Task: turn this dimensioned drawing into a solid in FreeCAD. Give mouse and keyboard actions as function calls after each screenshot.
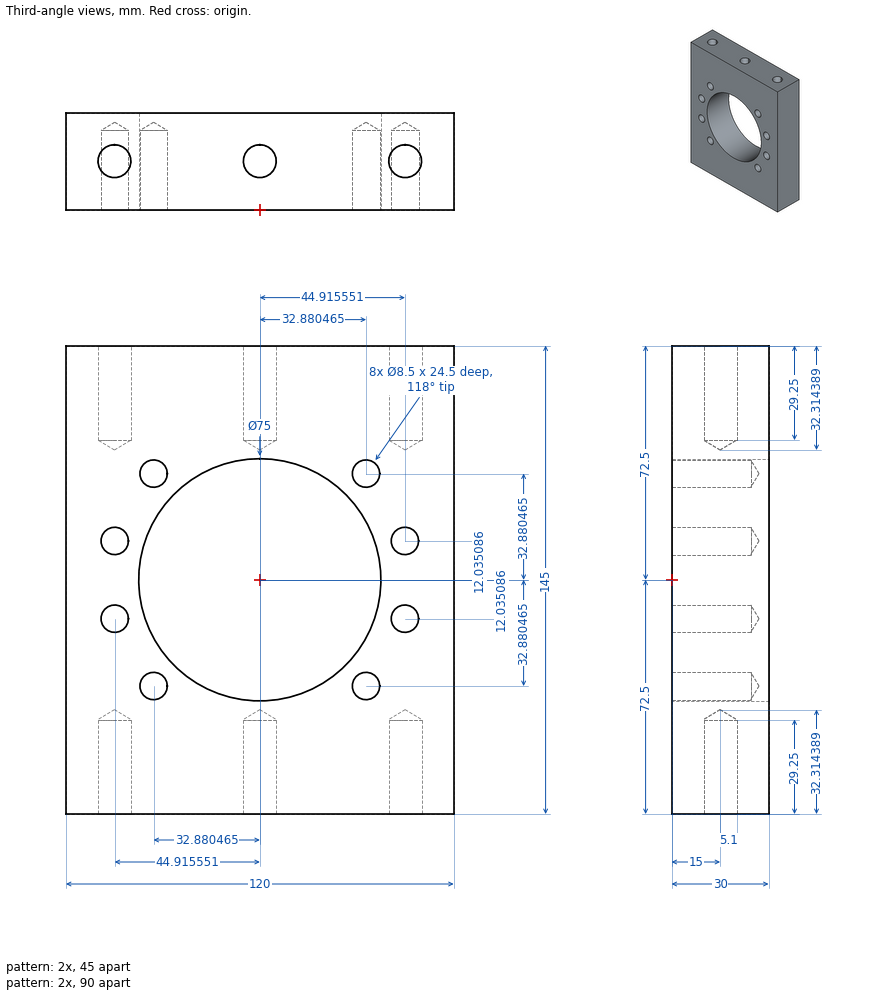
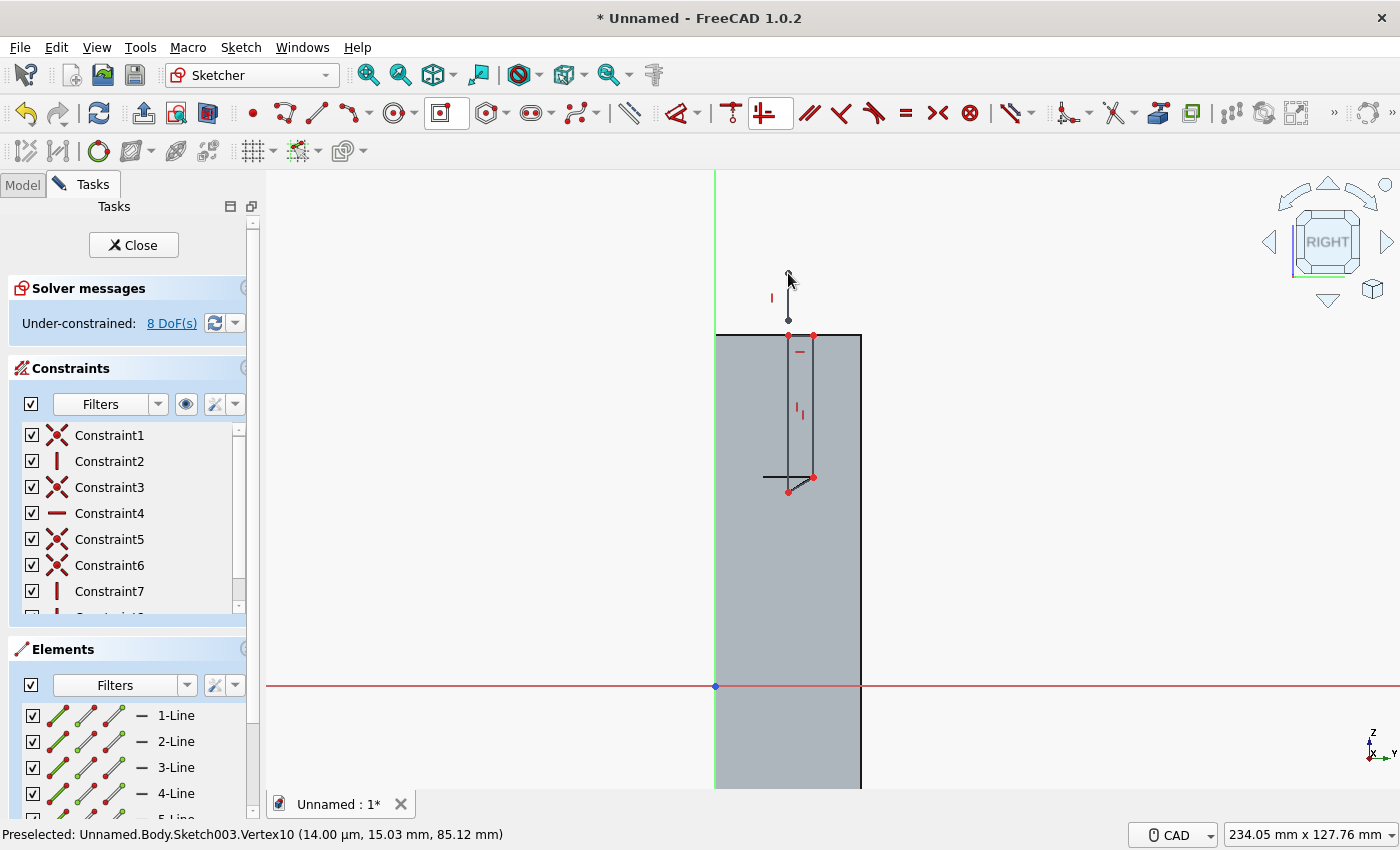
click(788, 307)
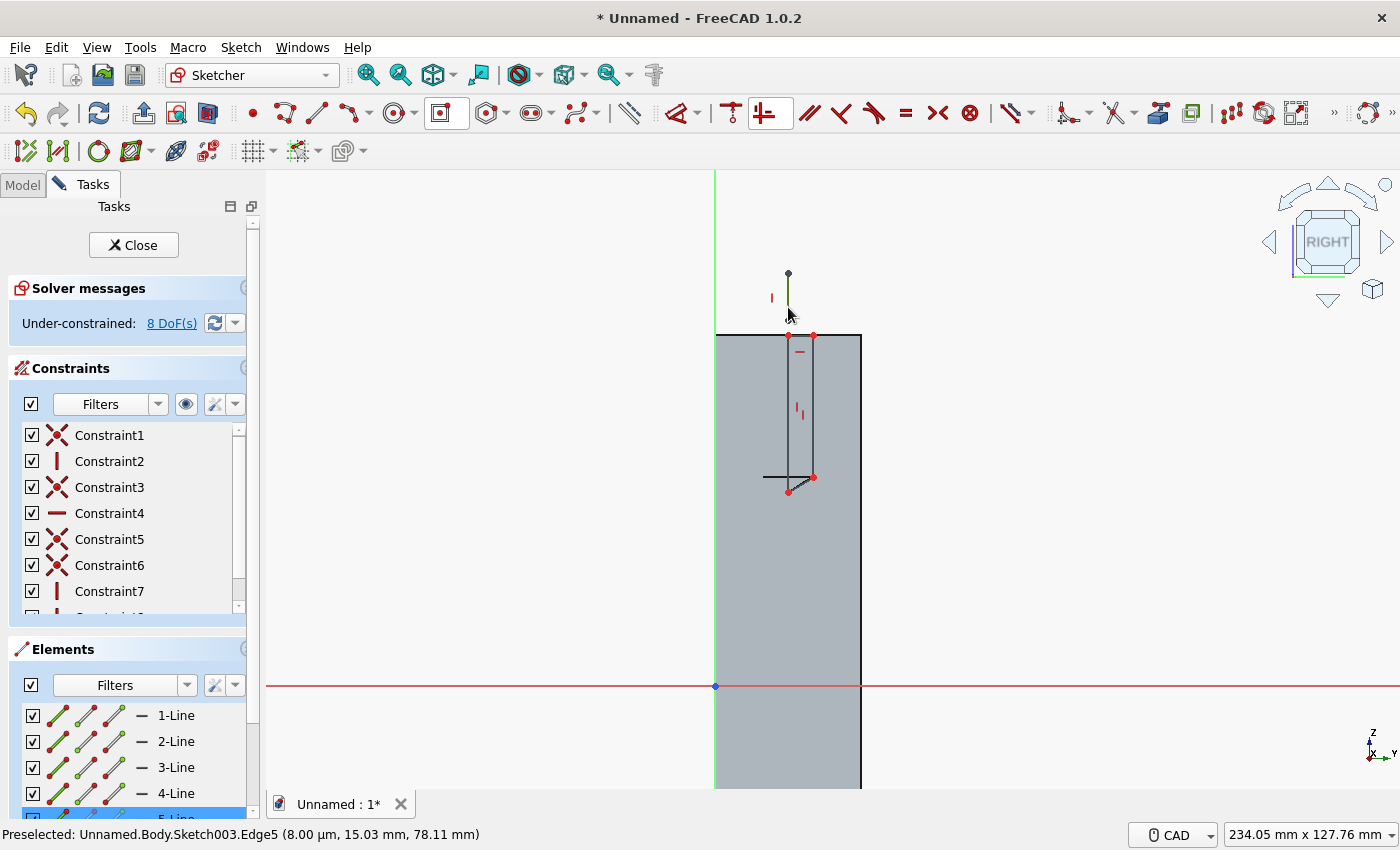
click(630, 114)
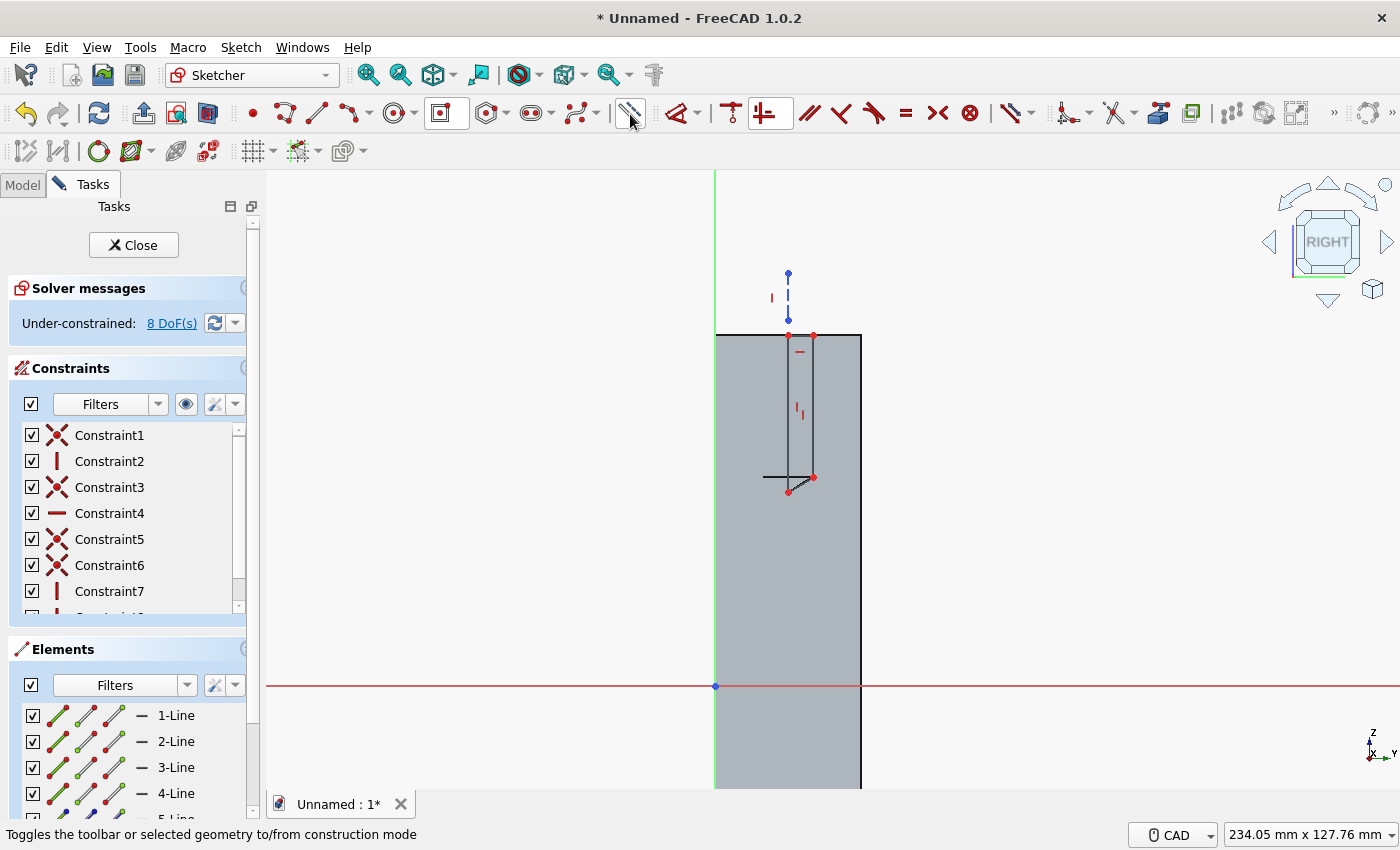
click(676, 114)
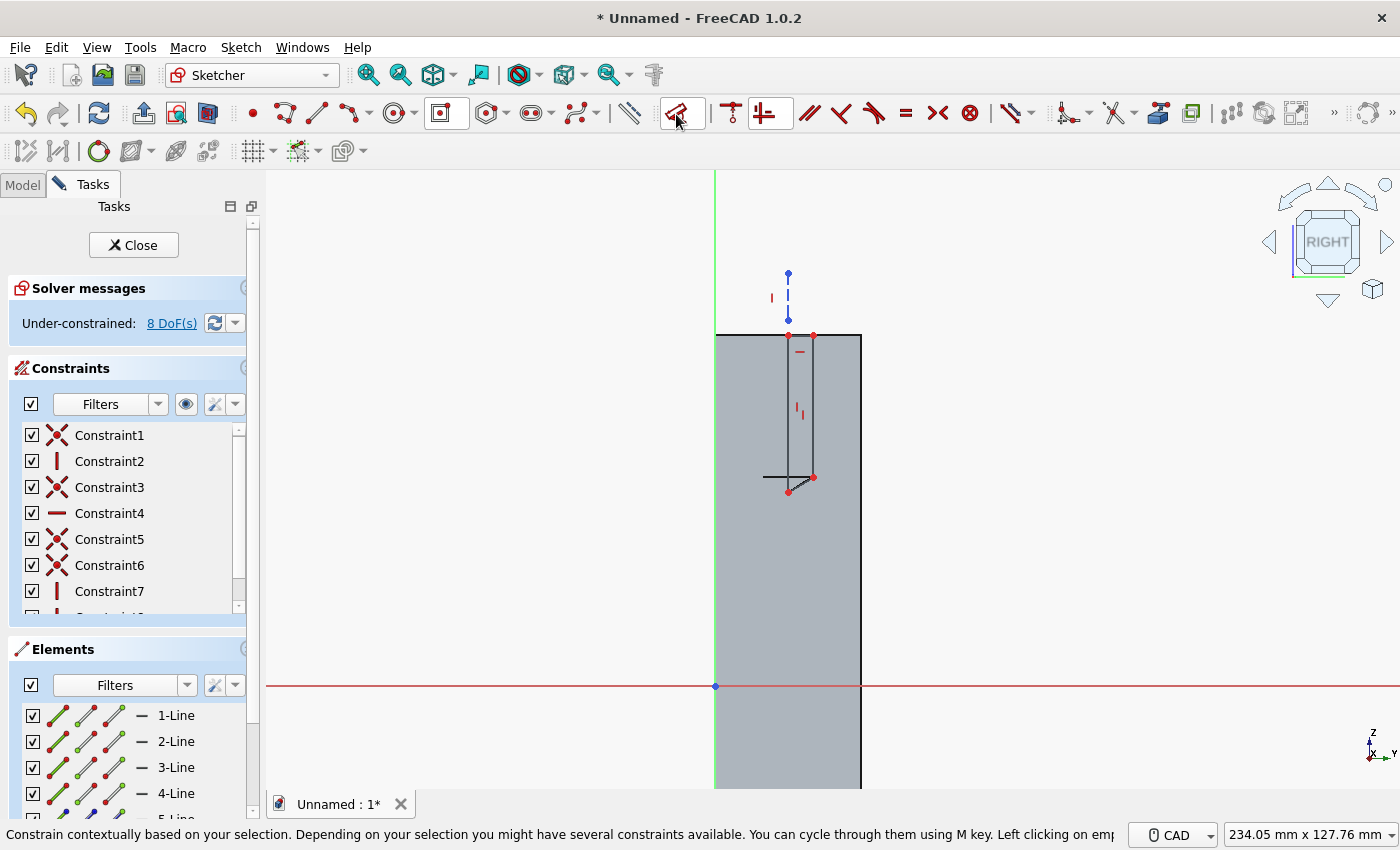
scroll(803, 336, up, 3)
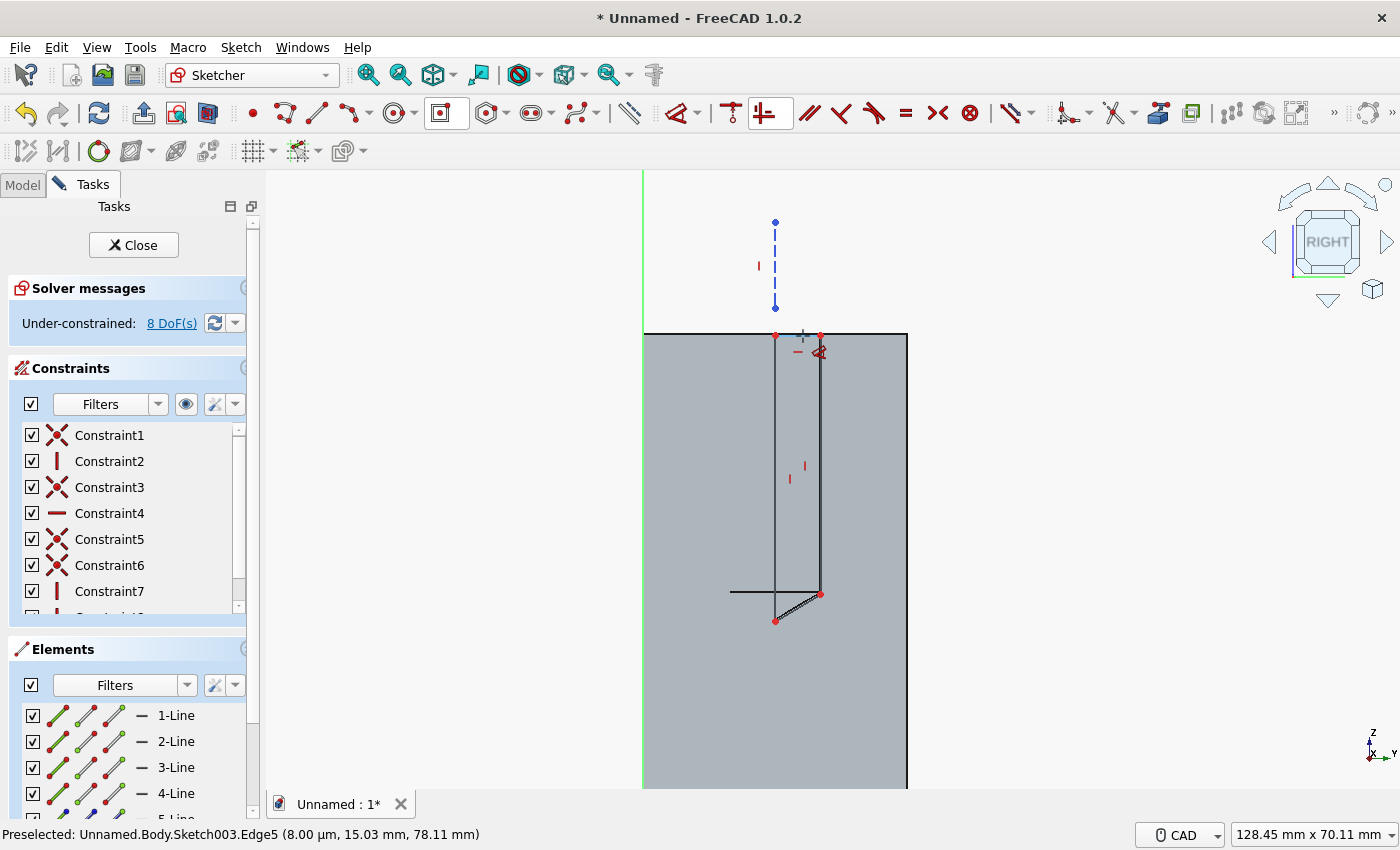
click(803, 336)
click(798, 302)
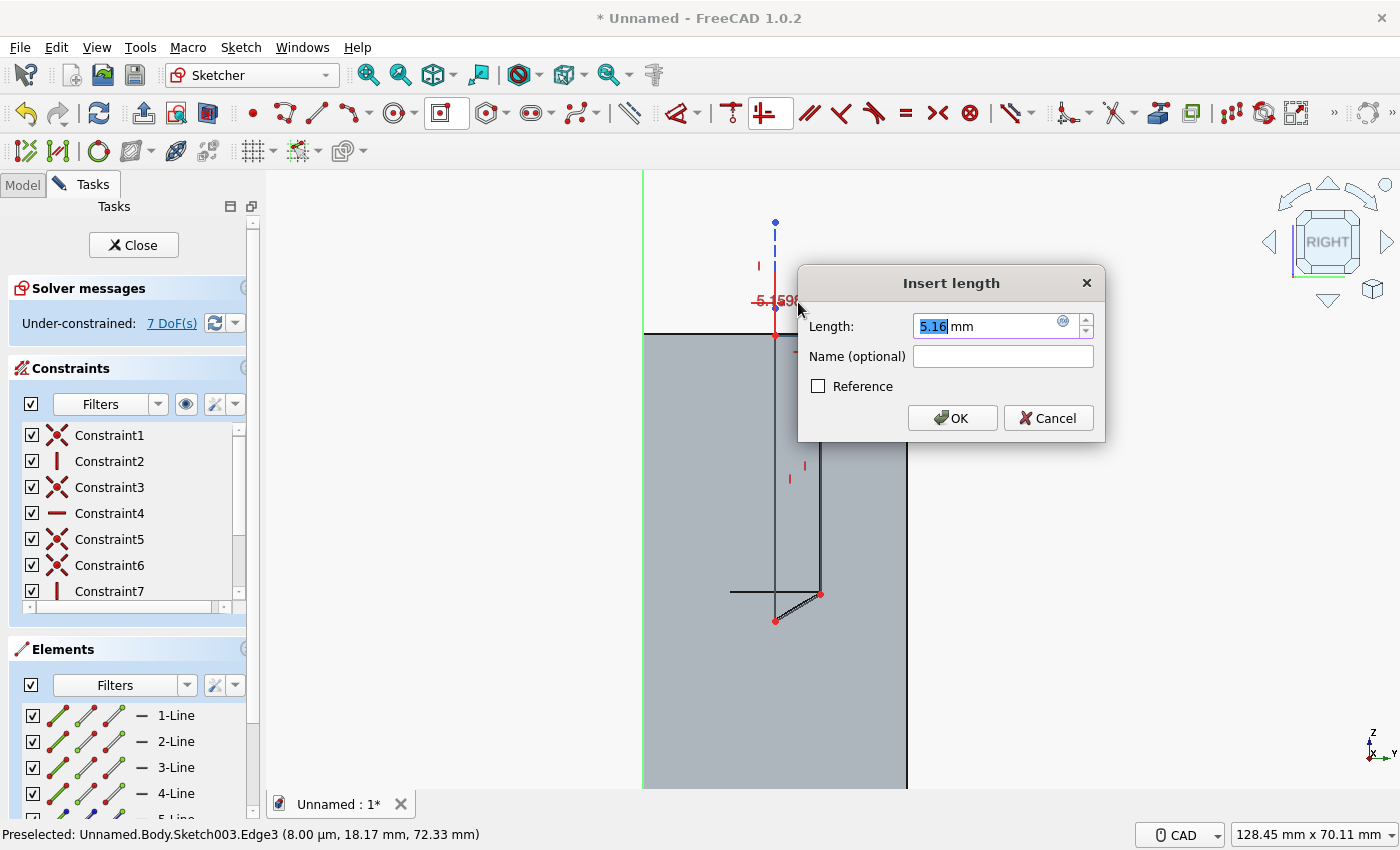
text(5.1)
key(Return)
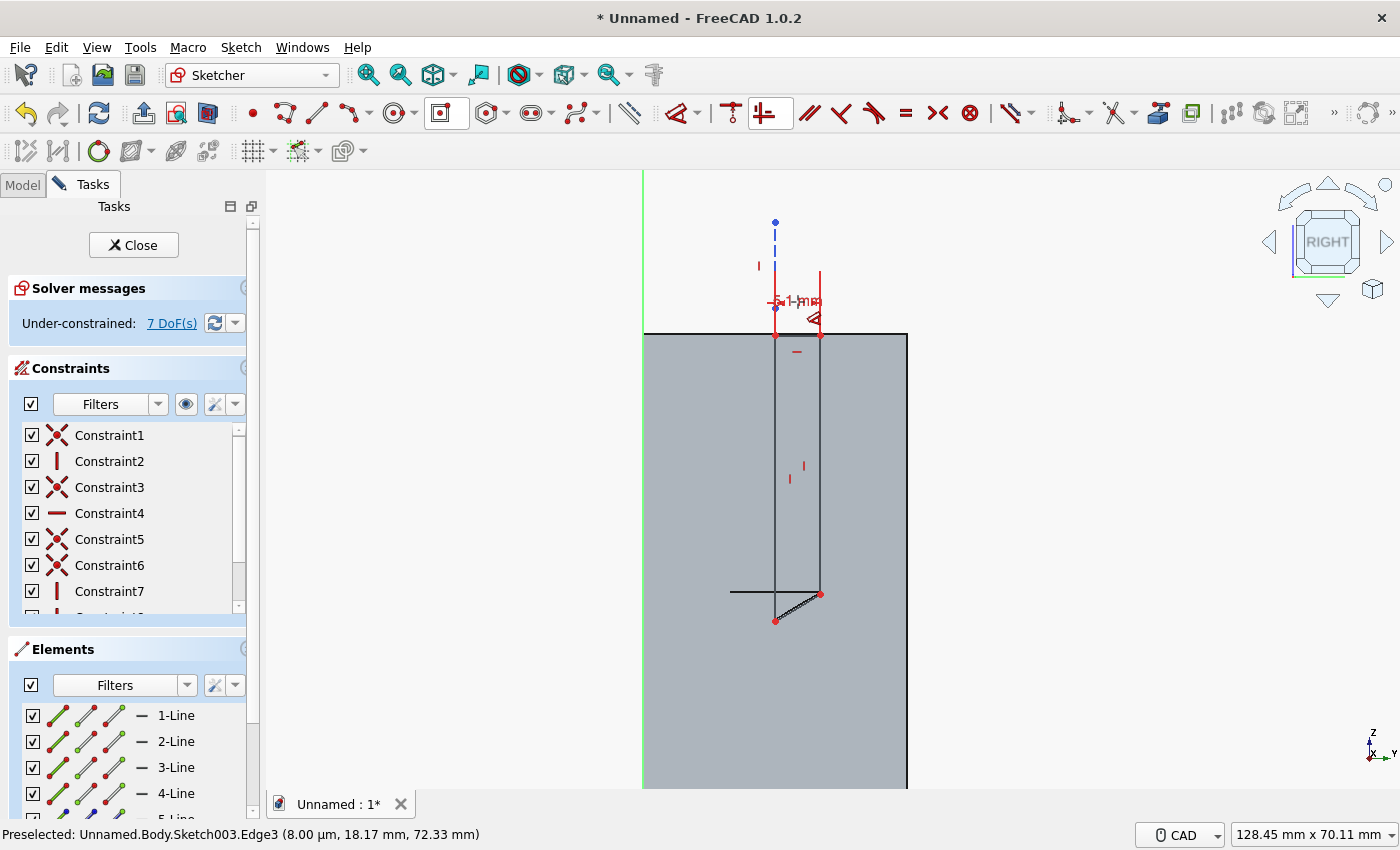
click(775, 622)
click(709, 588)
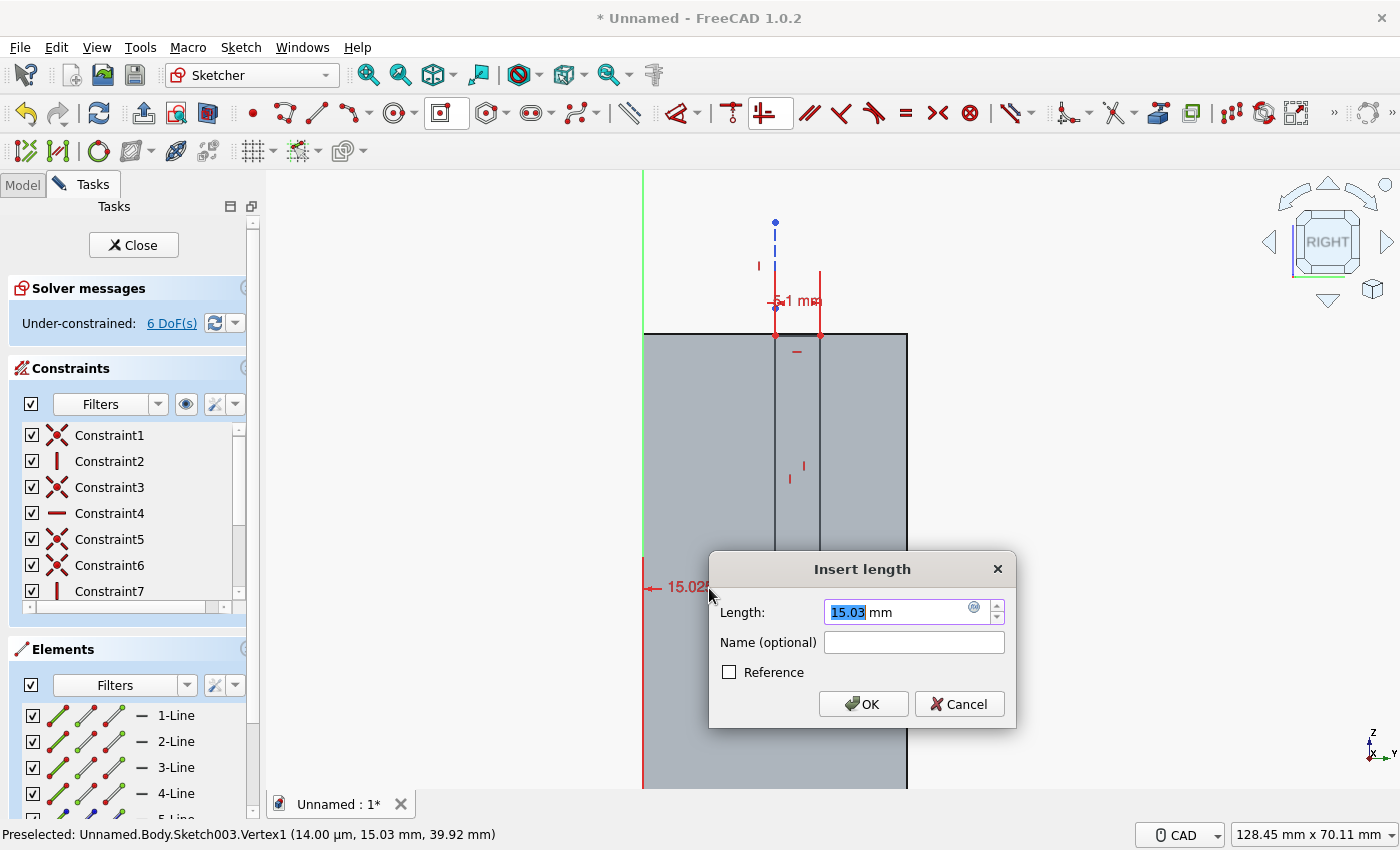
text(15)
key(Return)